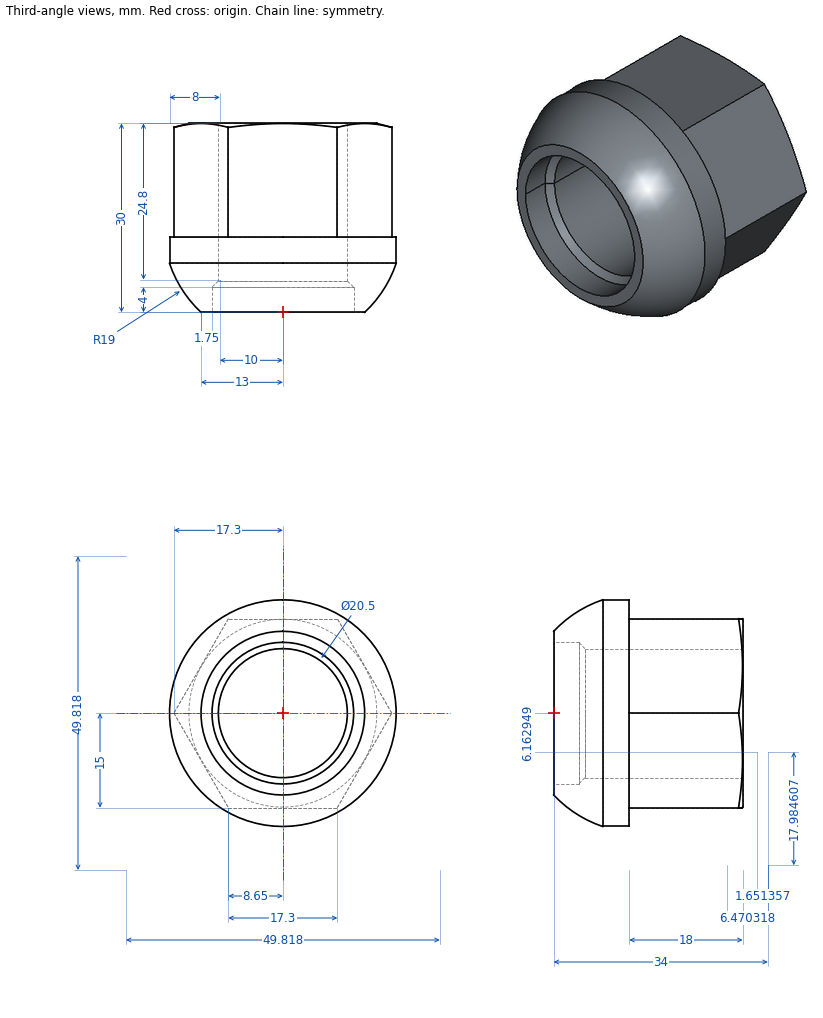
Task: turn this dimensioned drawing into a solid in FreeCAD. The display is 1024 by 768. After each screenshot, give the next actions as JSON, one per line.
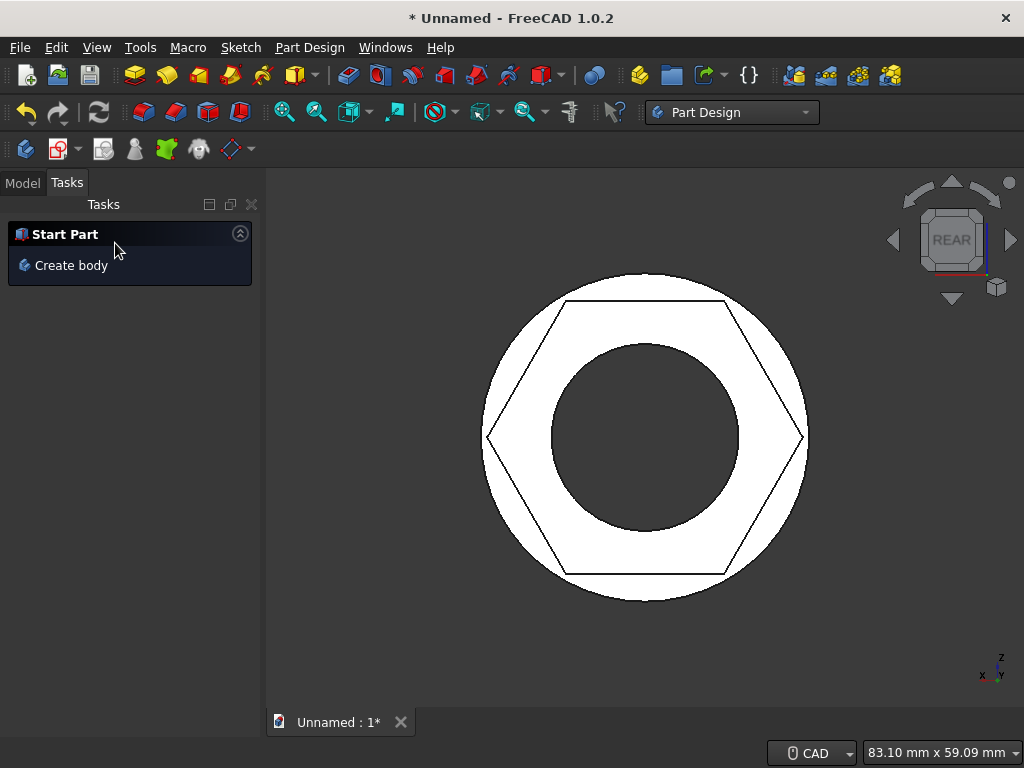
{"action": "left_click", "coordinate": [58, 150]}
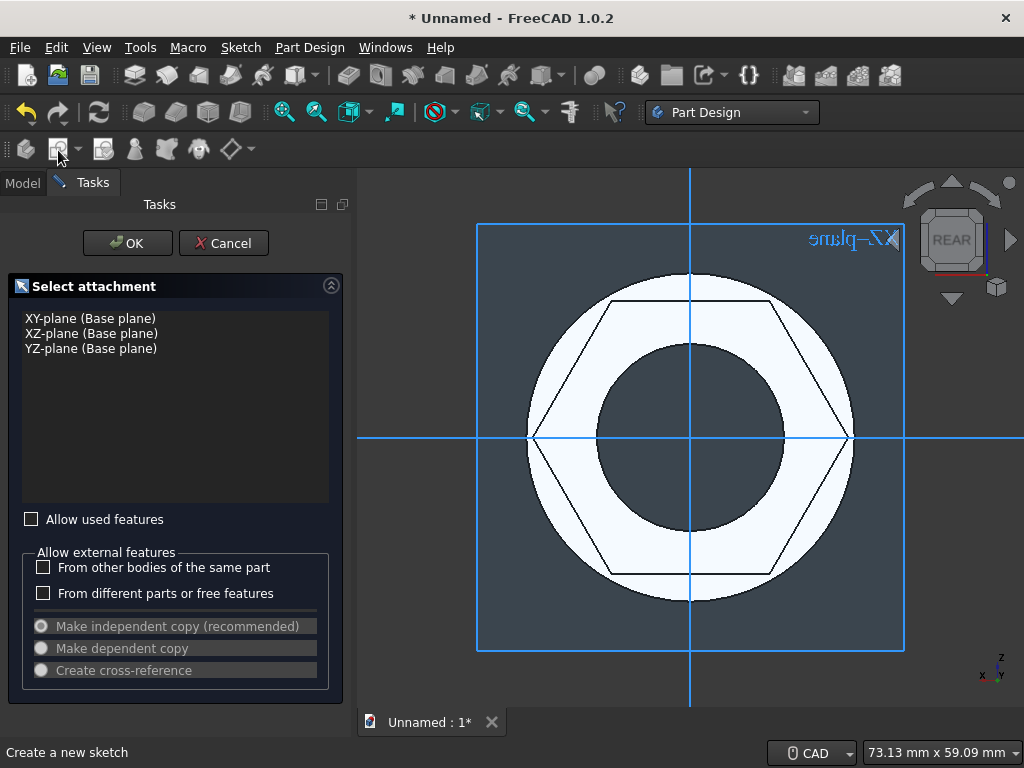
{"action": "left_click", "coordinate": [82, 348]}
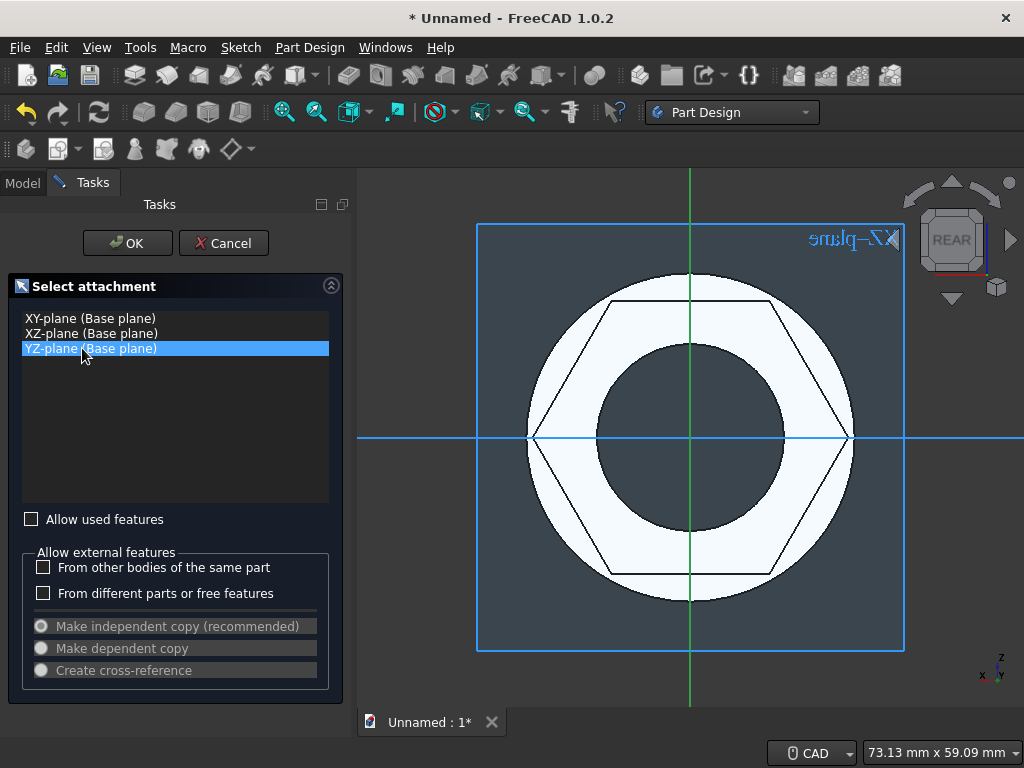
{"action": "left_click", "coordinate": [128, 243]}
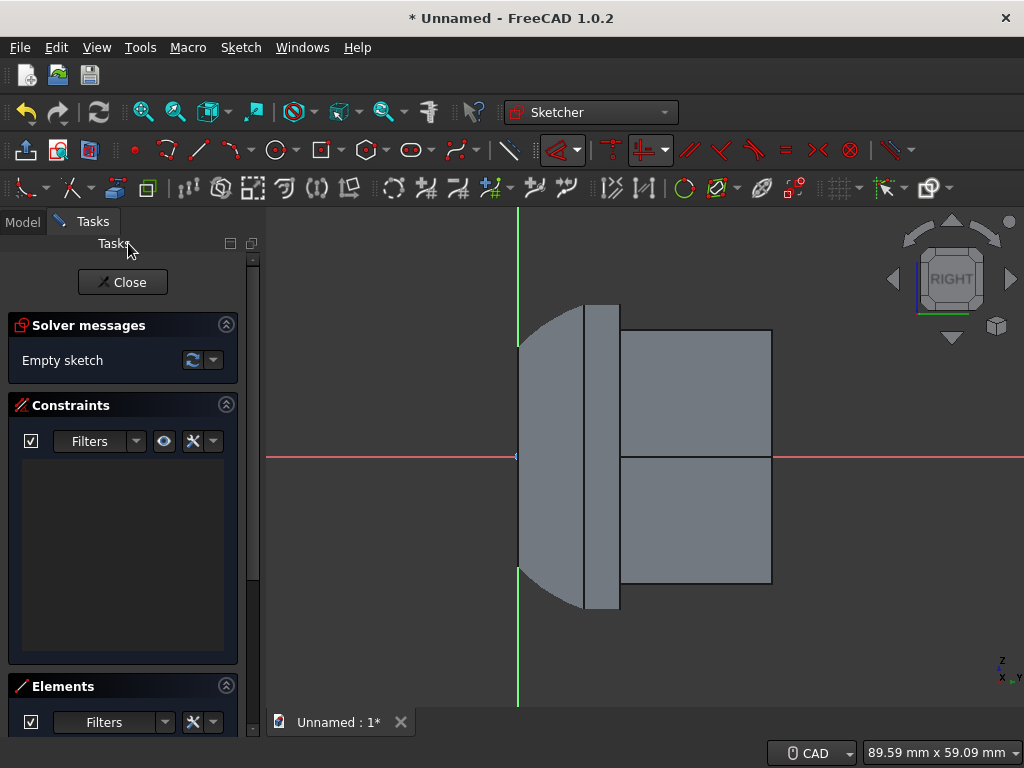
{"action": "key", "text": "q s"}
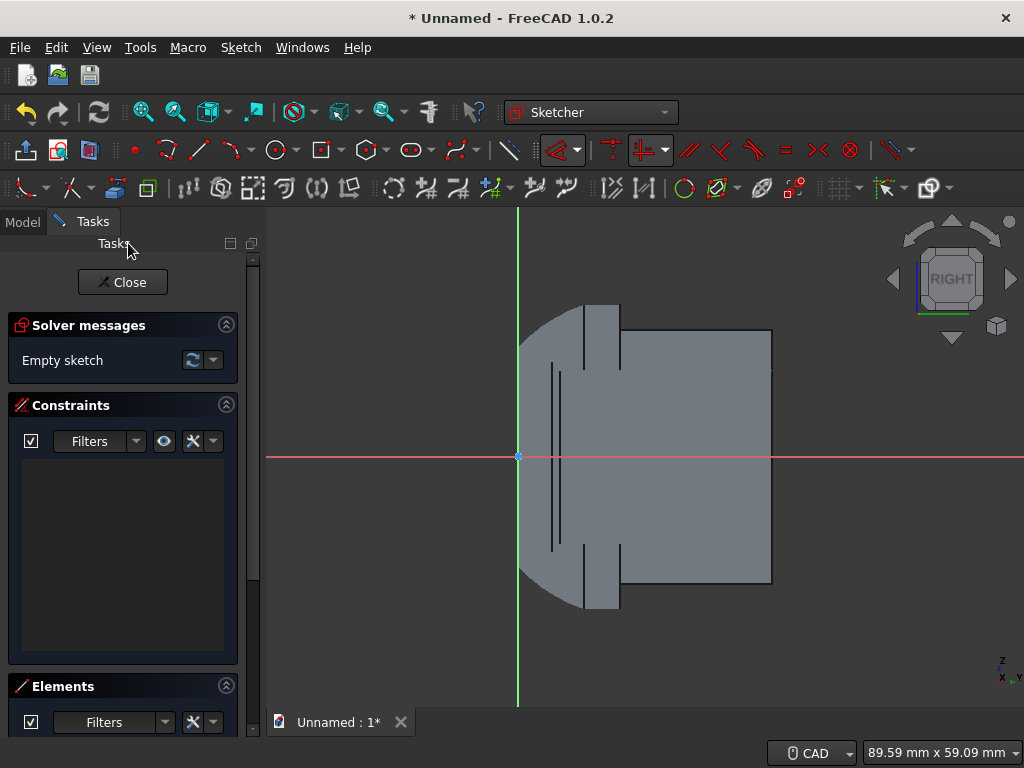
{"action": "scroll", "coordinate": [836, 679], "scroll_direction": "up", "scroll_amount": 2}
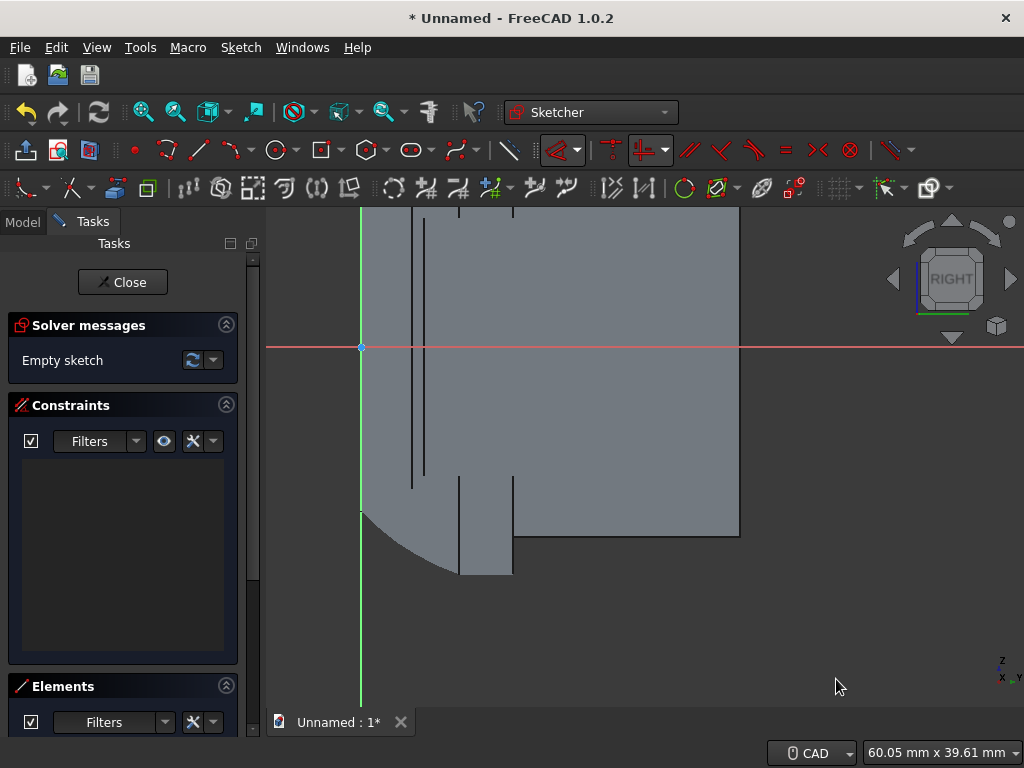
{"action": "key", "text": "g m"}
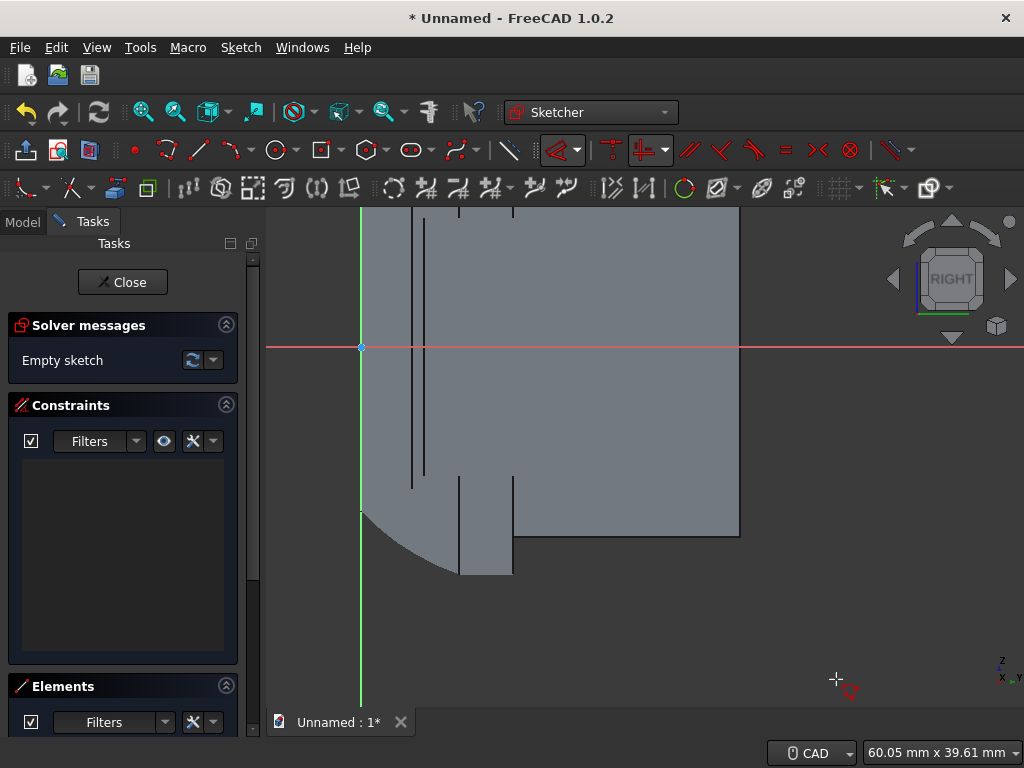
{"action": "left_click", "coordinate": [770, 425]}
{"action": "left_click", "coordinate": [709, 652]}
{"action": "left_click", "coordinate": [791, 652]}
{"action": "left_click", "coordinate": [791, 425]}
{"action": "left_click", "coordinate": [770, 426]}
{"action": "key", "text": "Escape"}
{"action": "key", "text": "Escape"}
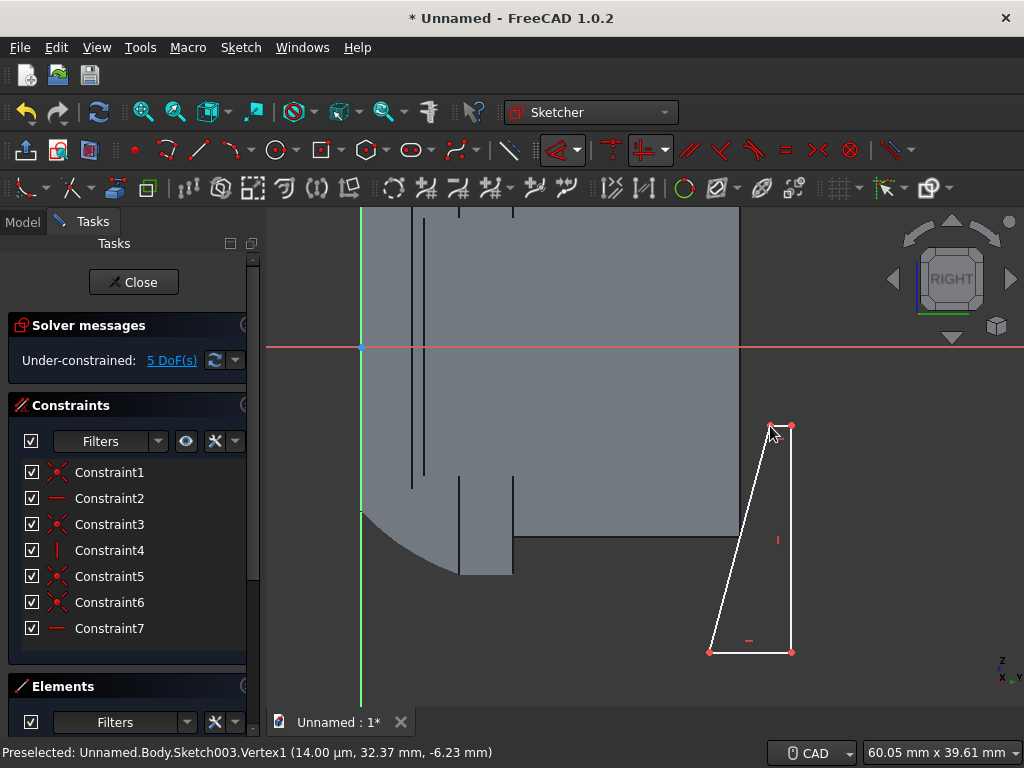
{"action": "left_click", "coordinate": [791, 653]}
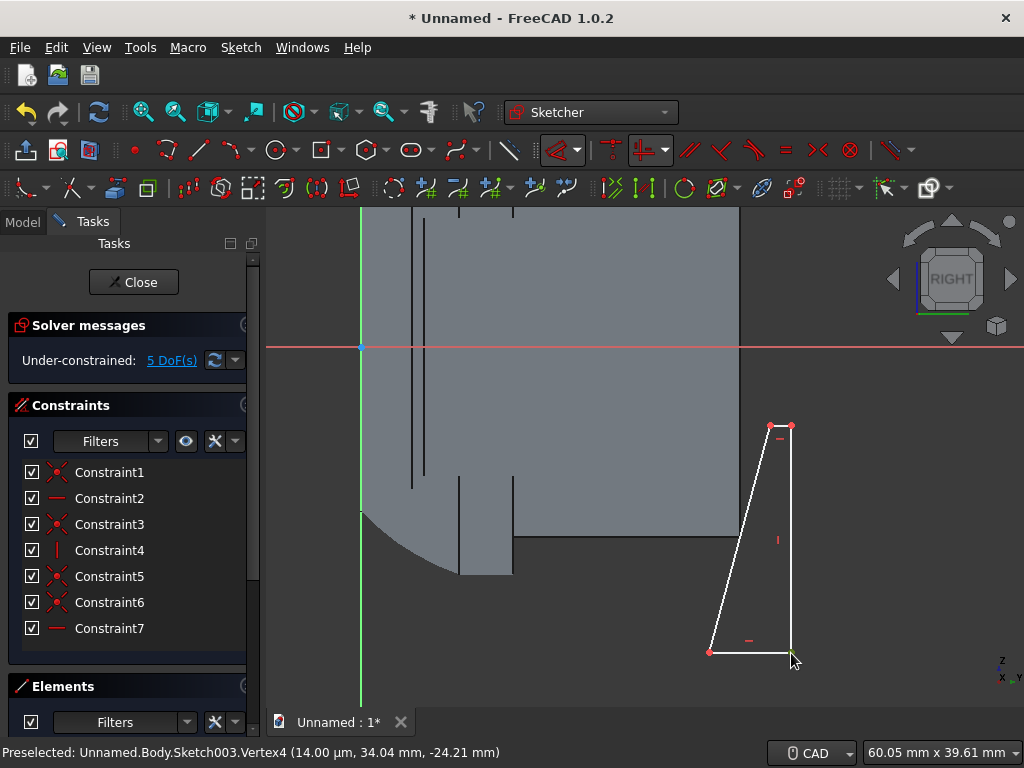
{"action": "key", "text": "l"}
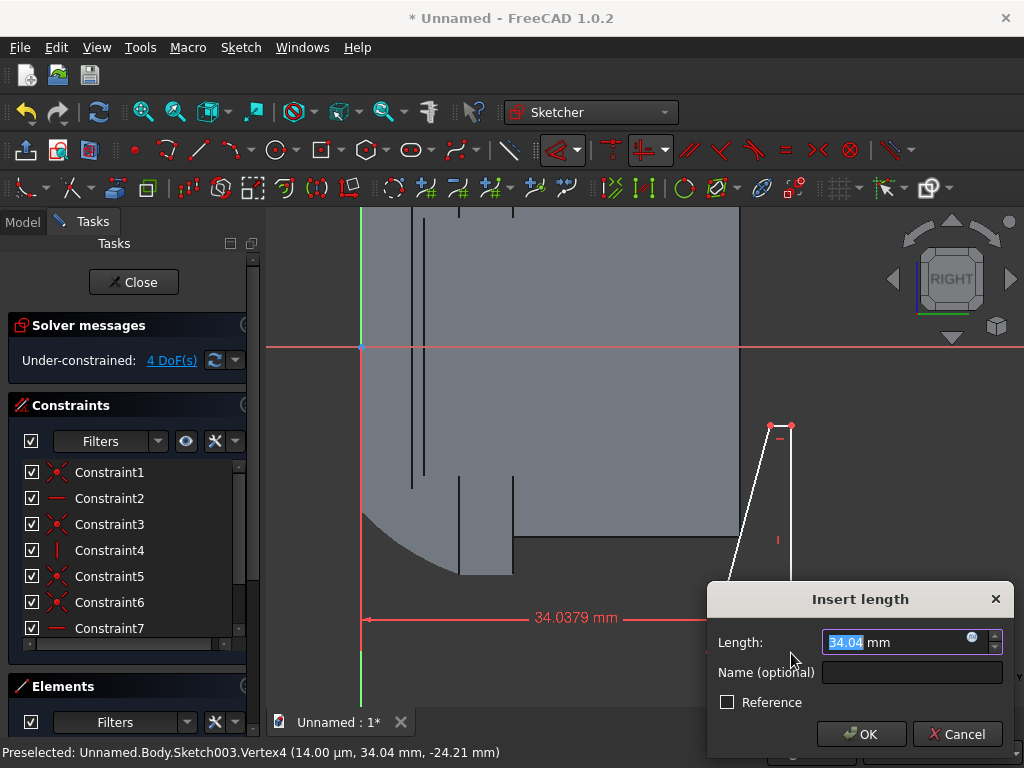
{"action": "type", "text": "34"}
{"action": "key", "text": "Return"}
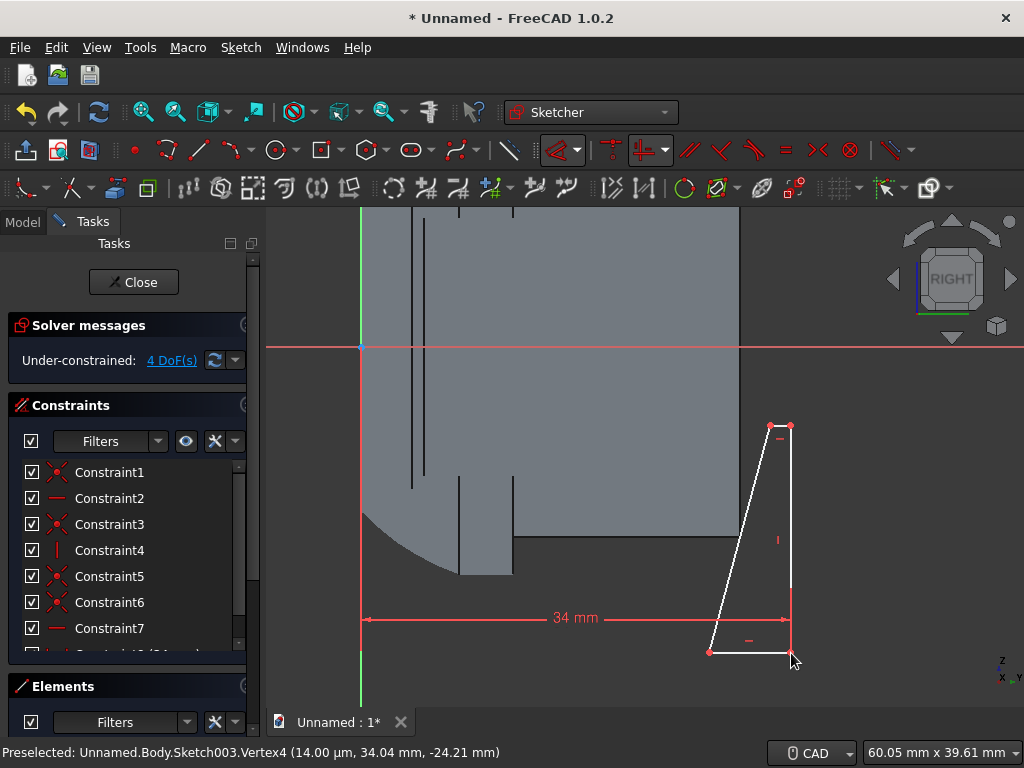
{"action": "left_click", "coordinate": [733, 653]}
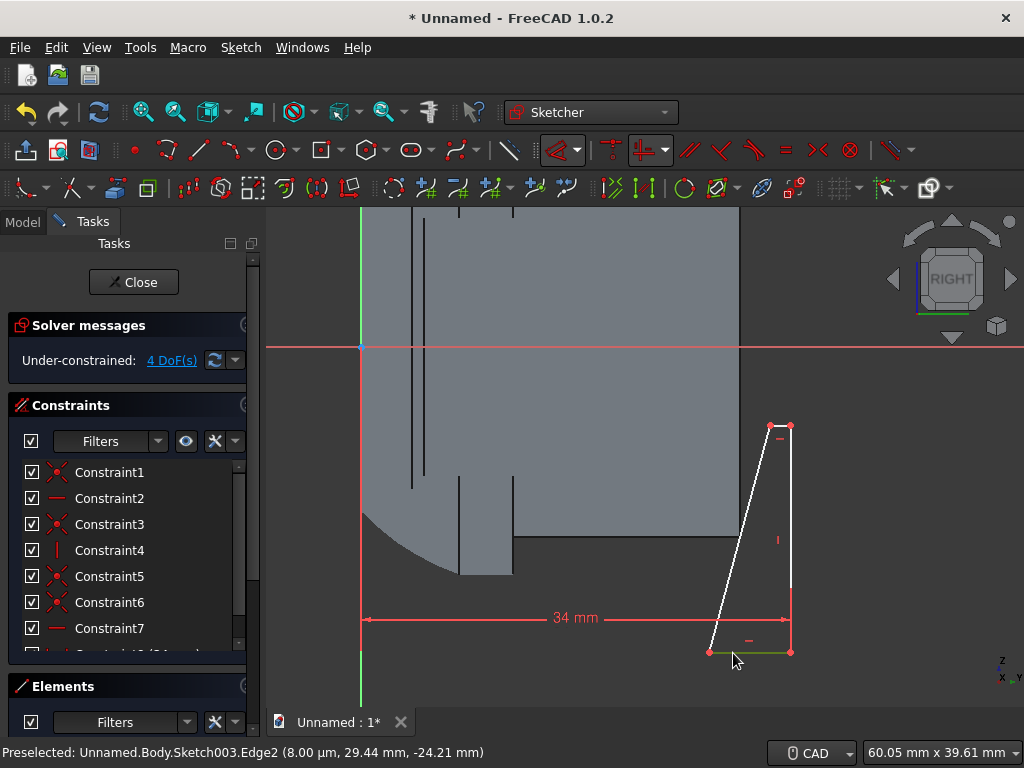
{"action": "key", "text": "l"}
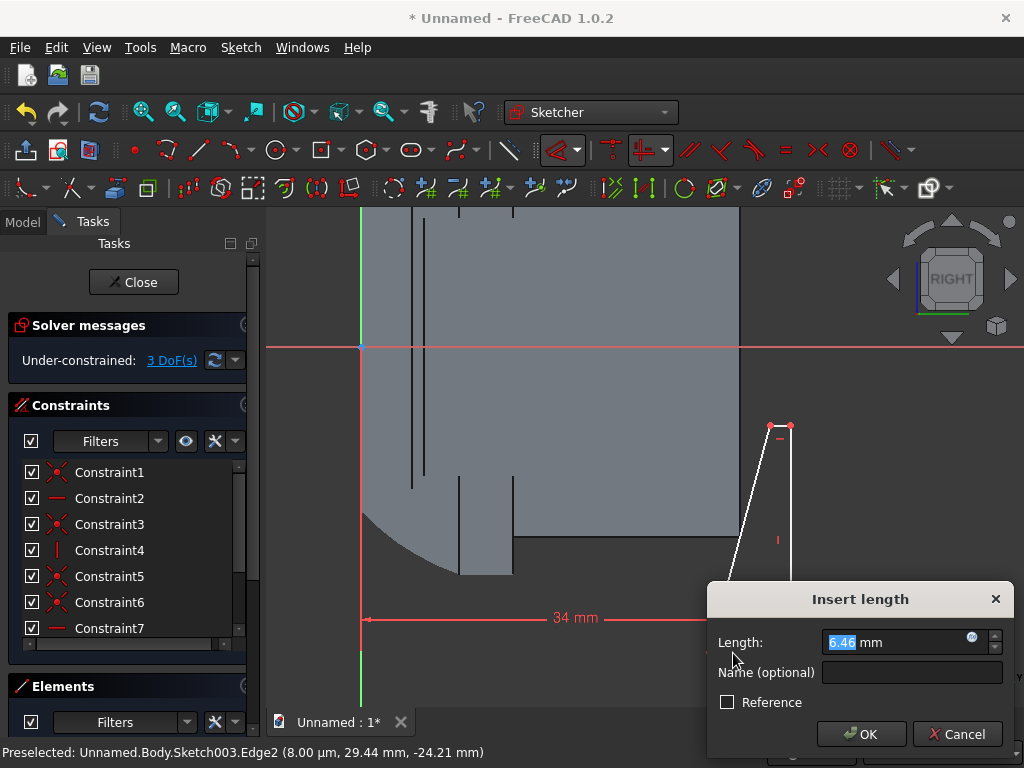
{"action": "type", "text": "6.470318"}
{"action": "key", "text": "Return"}